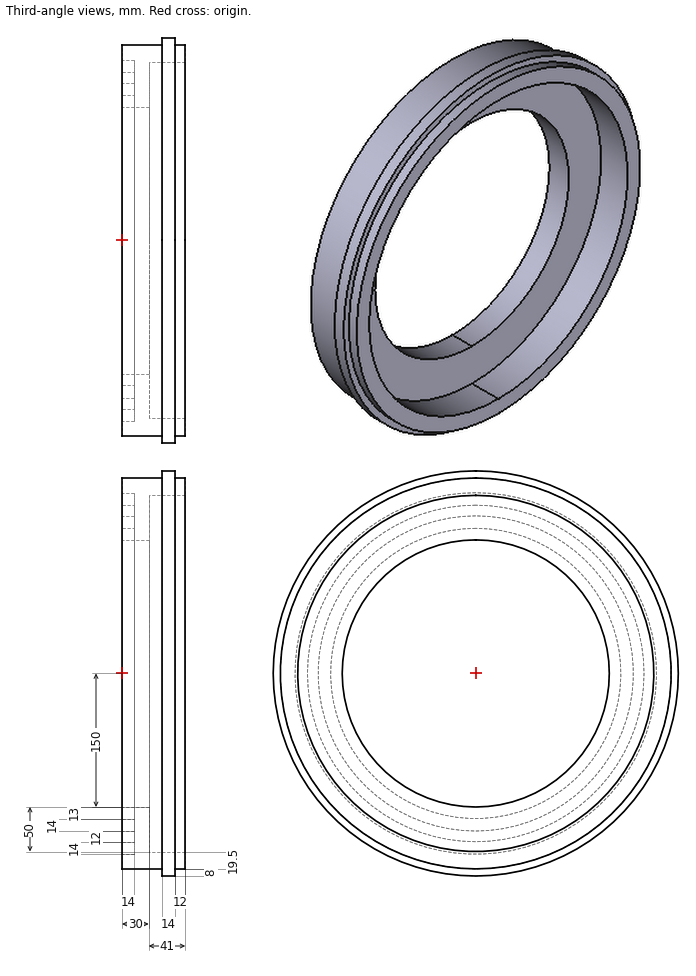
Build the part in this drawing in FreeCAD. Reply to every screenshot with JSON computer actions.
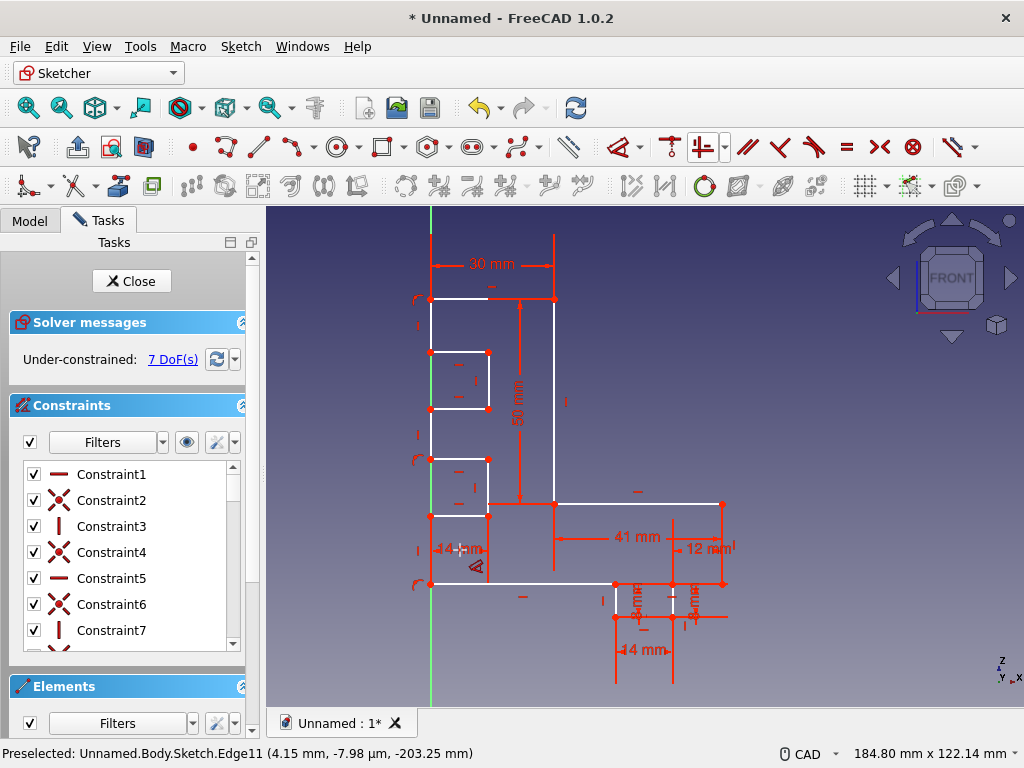
{"action": "left_click", "coordinate": [488, 499]}
{"action": "left_click", "coordinate": [454, 488]}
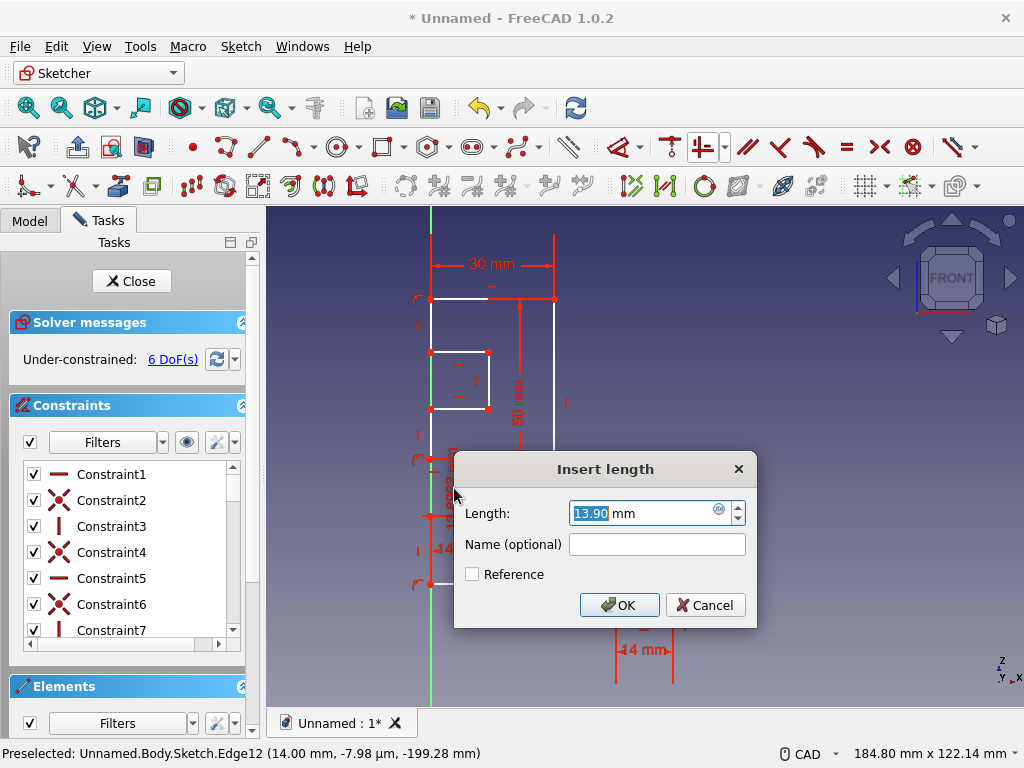
{"action": "type", "text": "14"}
{"action": "key", "text": "Return"}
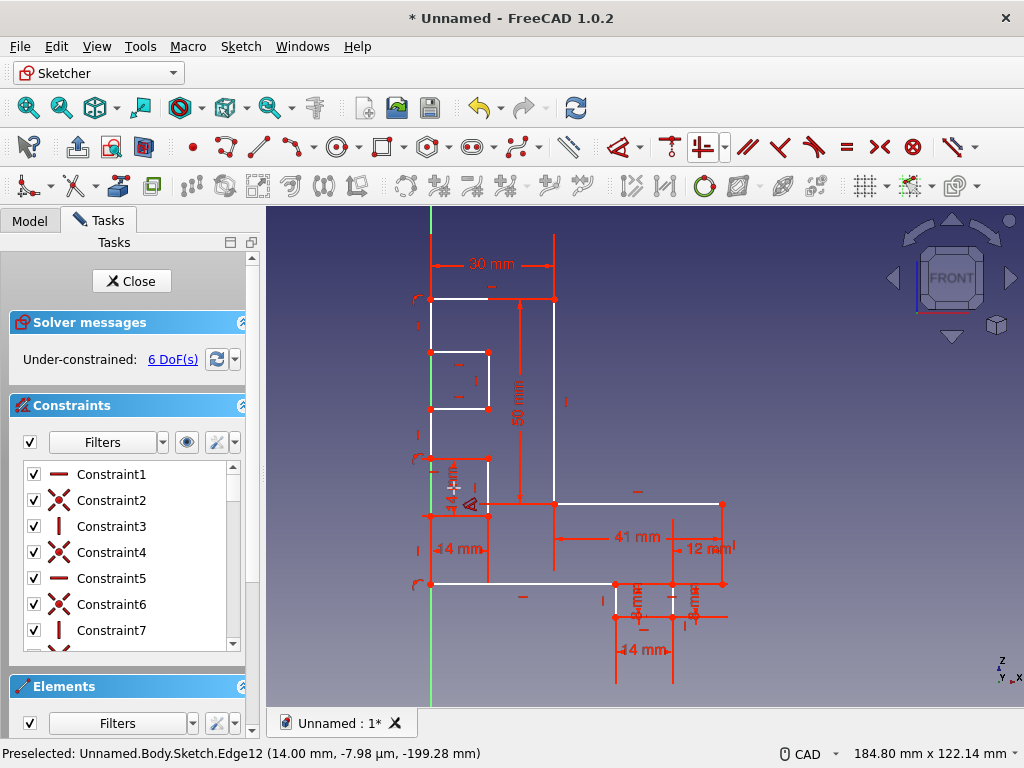
{"action": "left_click", "coordinate": [431, 444]}
{"action": "left_click", "coordinate": [397, 434]}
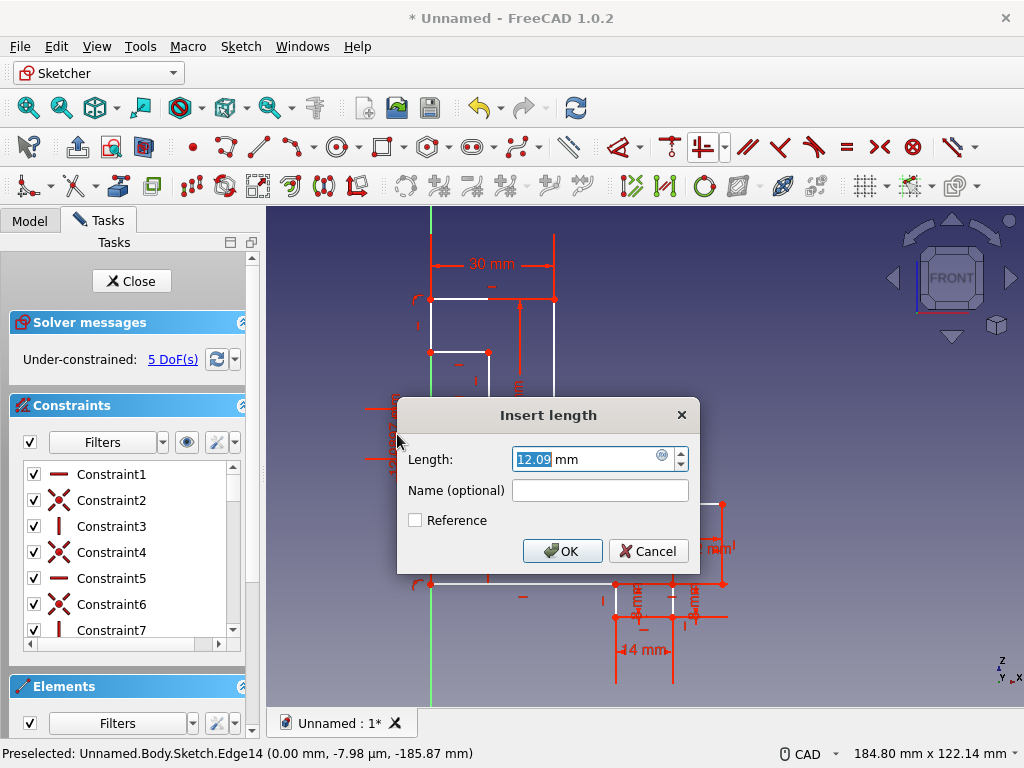
{"action": "type", "text": "12"}
{"action": "key", "text": "Return"}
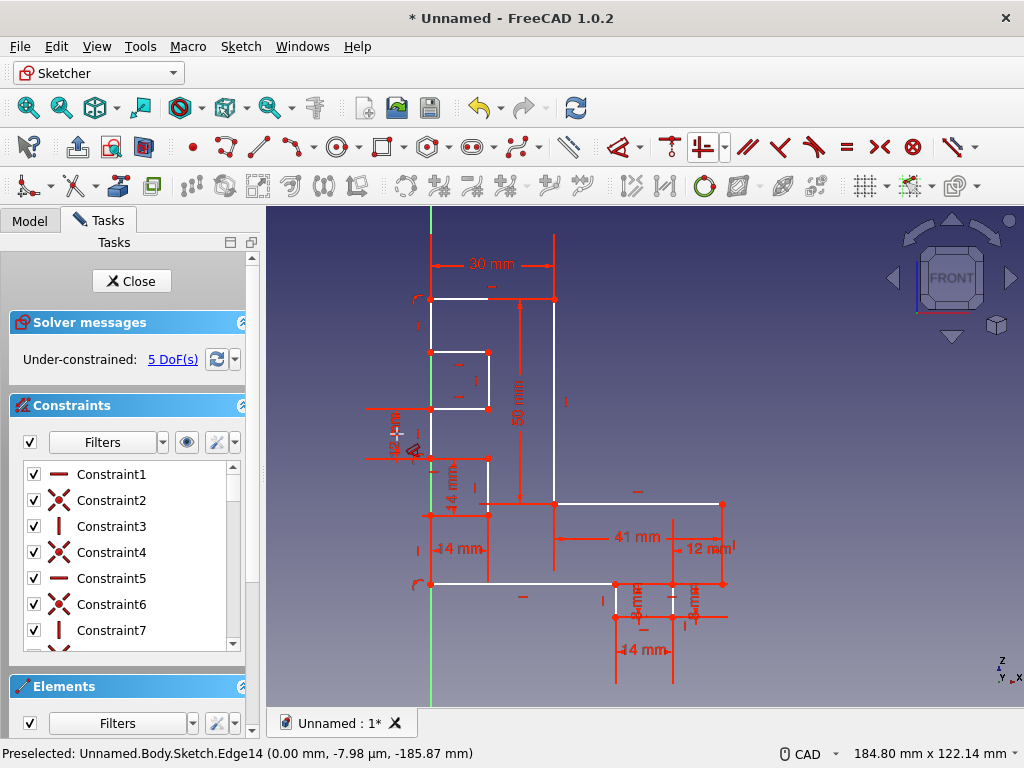
{"action": "left_click", "coordinate": [448, 409]}
{"action": "left_click", "coordinate": [460, 375]}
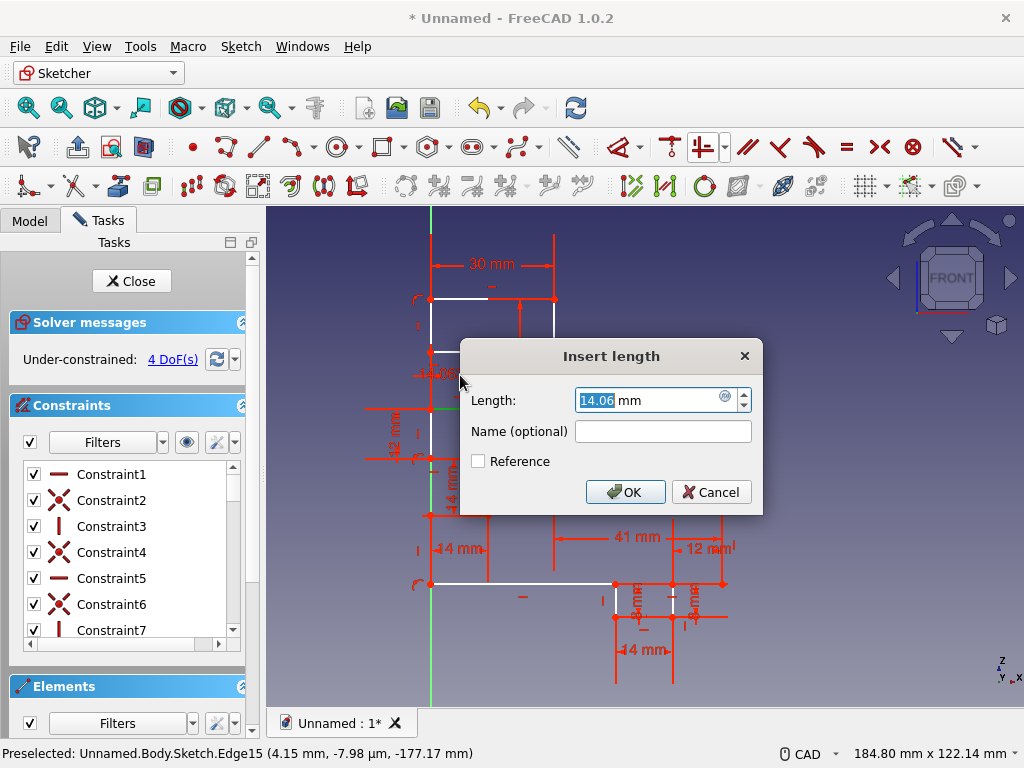
{"action": "type", "text": "14"}
{"action": "key", "text": "Return"}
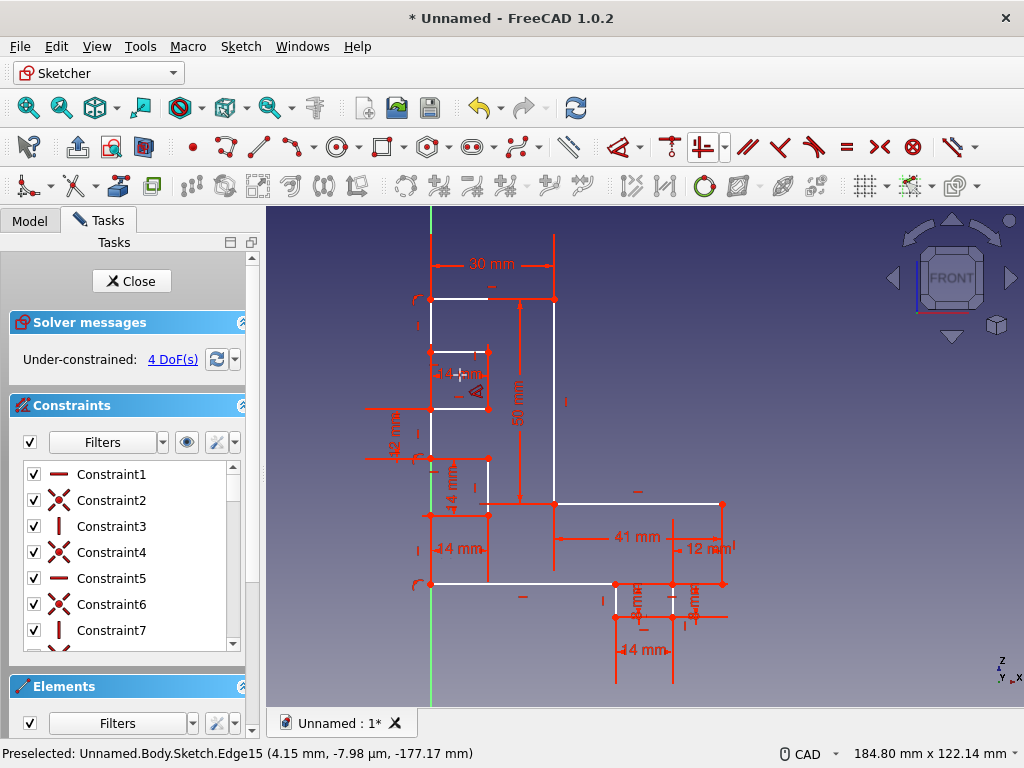
{"action": "left_click", "coordinate": [488, 392]}
{"action": "left_click", "coordinate": [406, 401]}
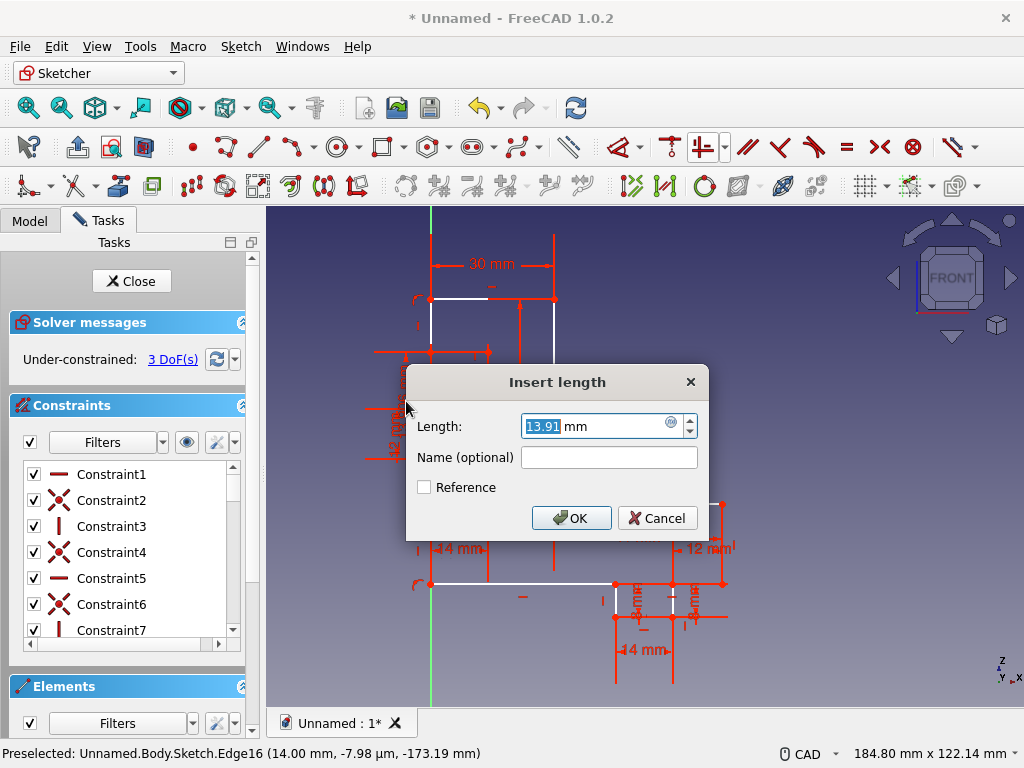
{"action": "type", "text": "14"}
{"action": "key", "text": "Return"}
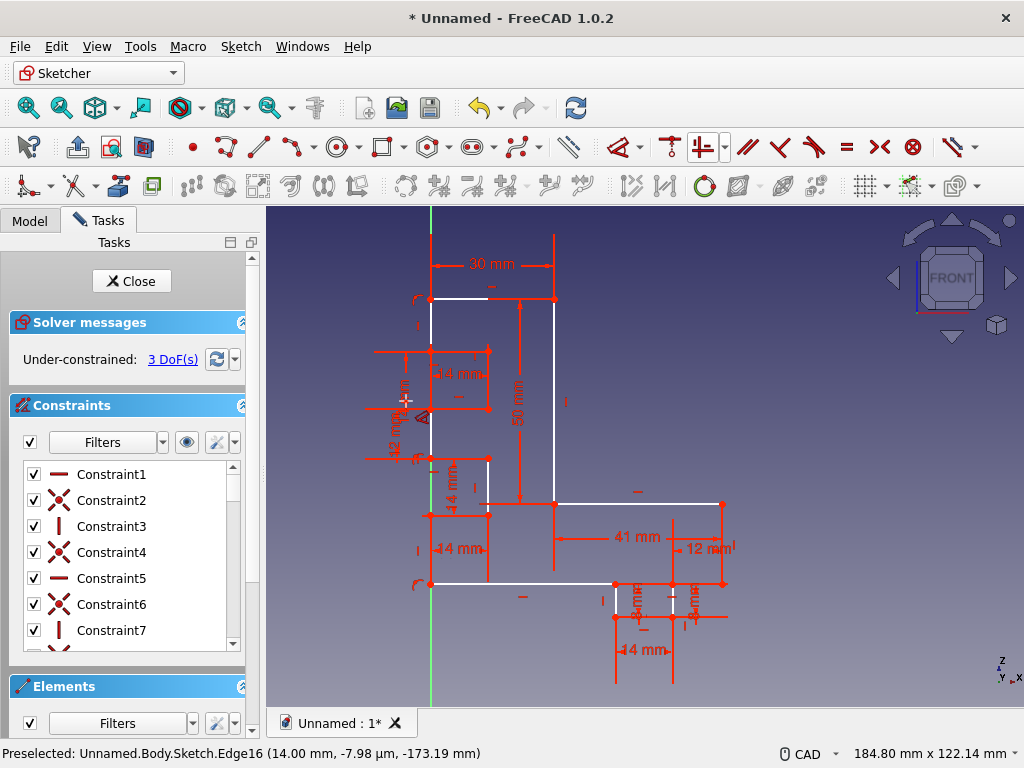
{"action": "left_click", "coordinate": [431, 336]}
{"action": "left_click", "coordinate": [397, 326]}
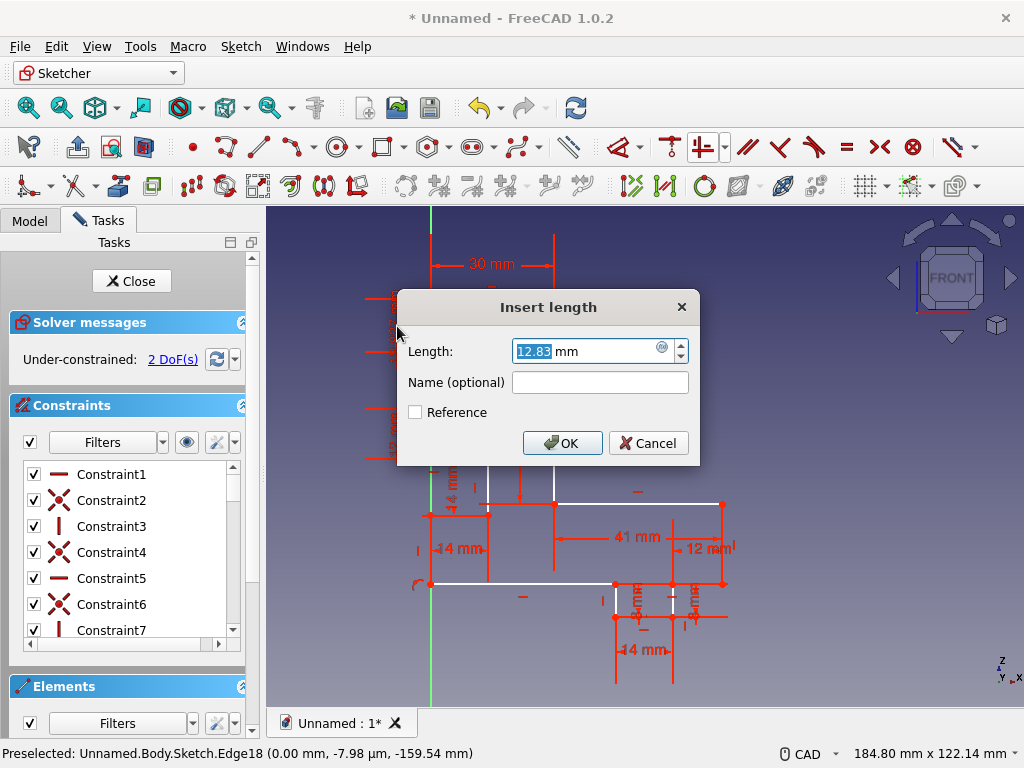
{"action": "type", "text": "13"}
{"action": "key", "text": "Return"}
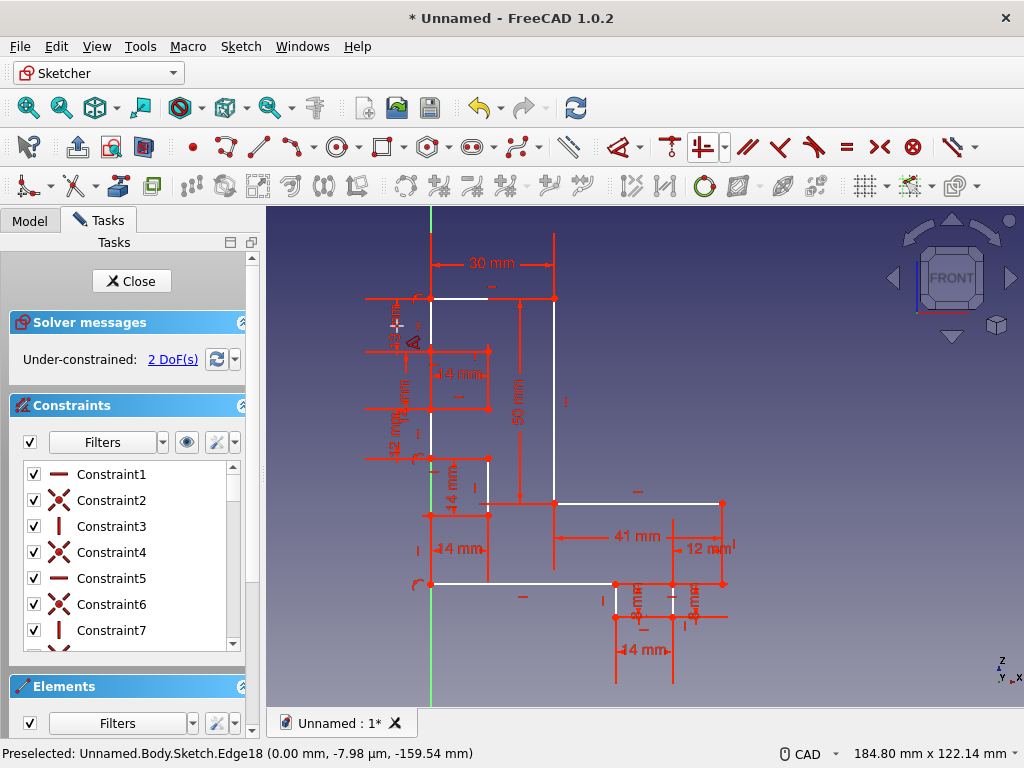
{"action": "left_click", "coordinate": [722, 528]}
{"action": "left_click", "coordinate": [756, 525]}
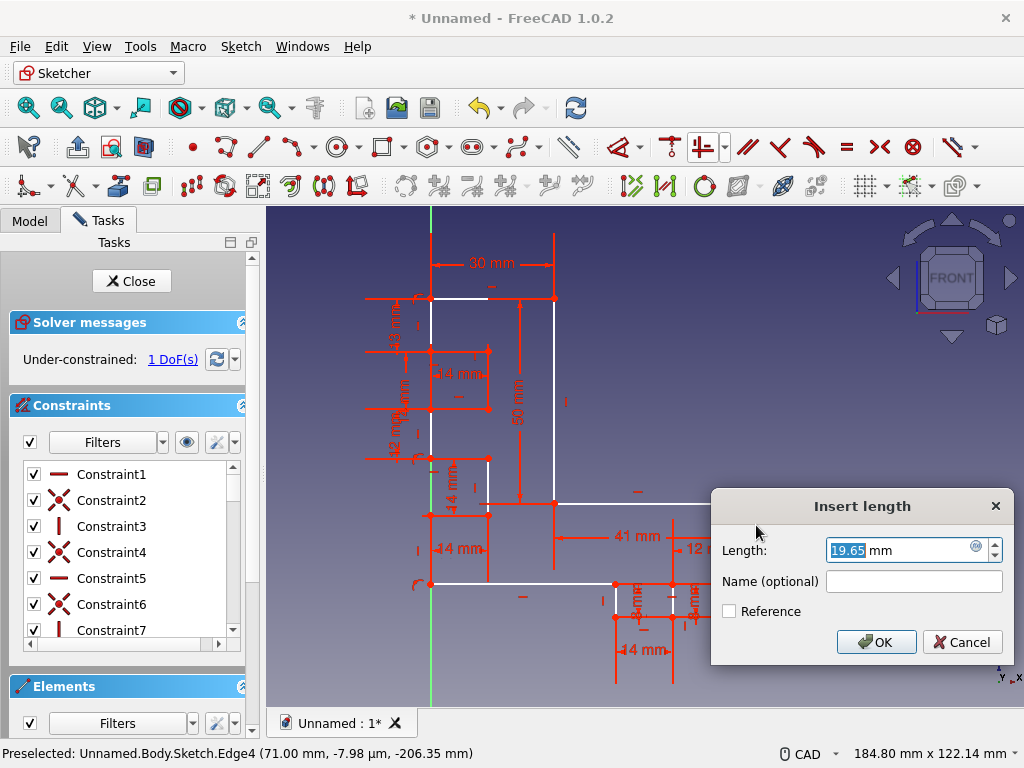
{"action": "type", "text": "19.5"}
{"action": "key", "text": "Return"}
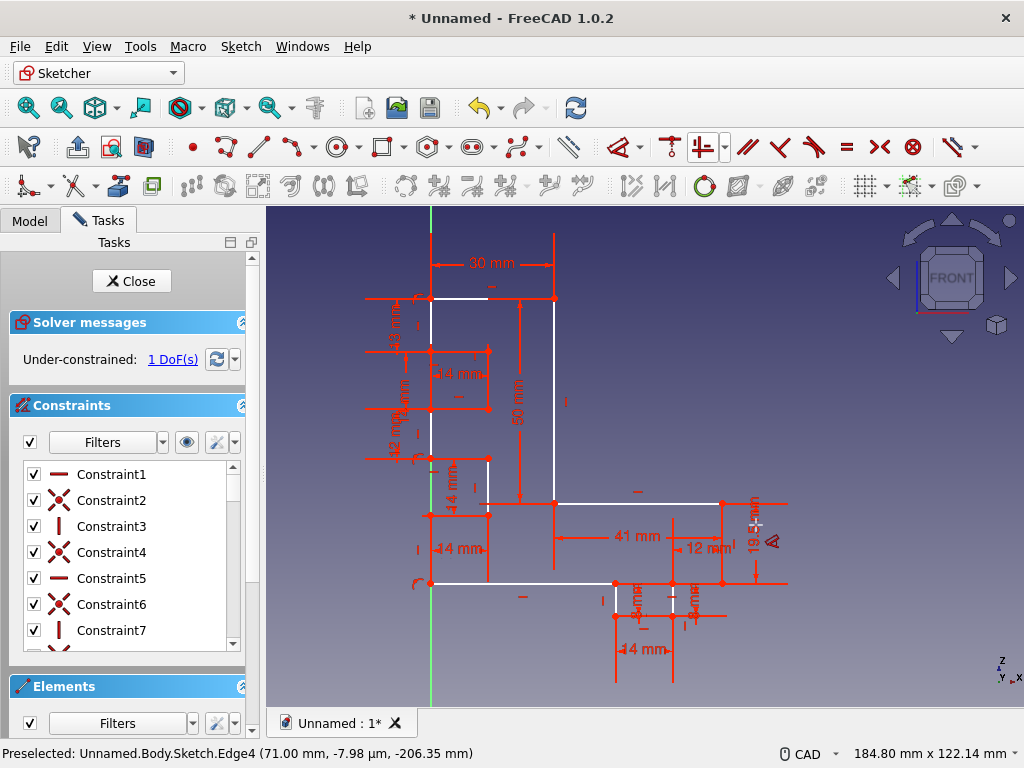
{"action": "left_click", "coordinate": [431, 299]}
{"action": "left_click", "coordinate": [397, 266]}